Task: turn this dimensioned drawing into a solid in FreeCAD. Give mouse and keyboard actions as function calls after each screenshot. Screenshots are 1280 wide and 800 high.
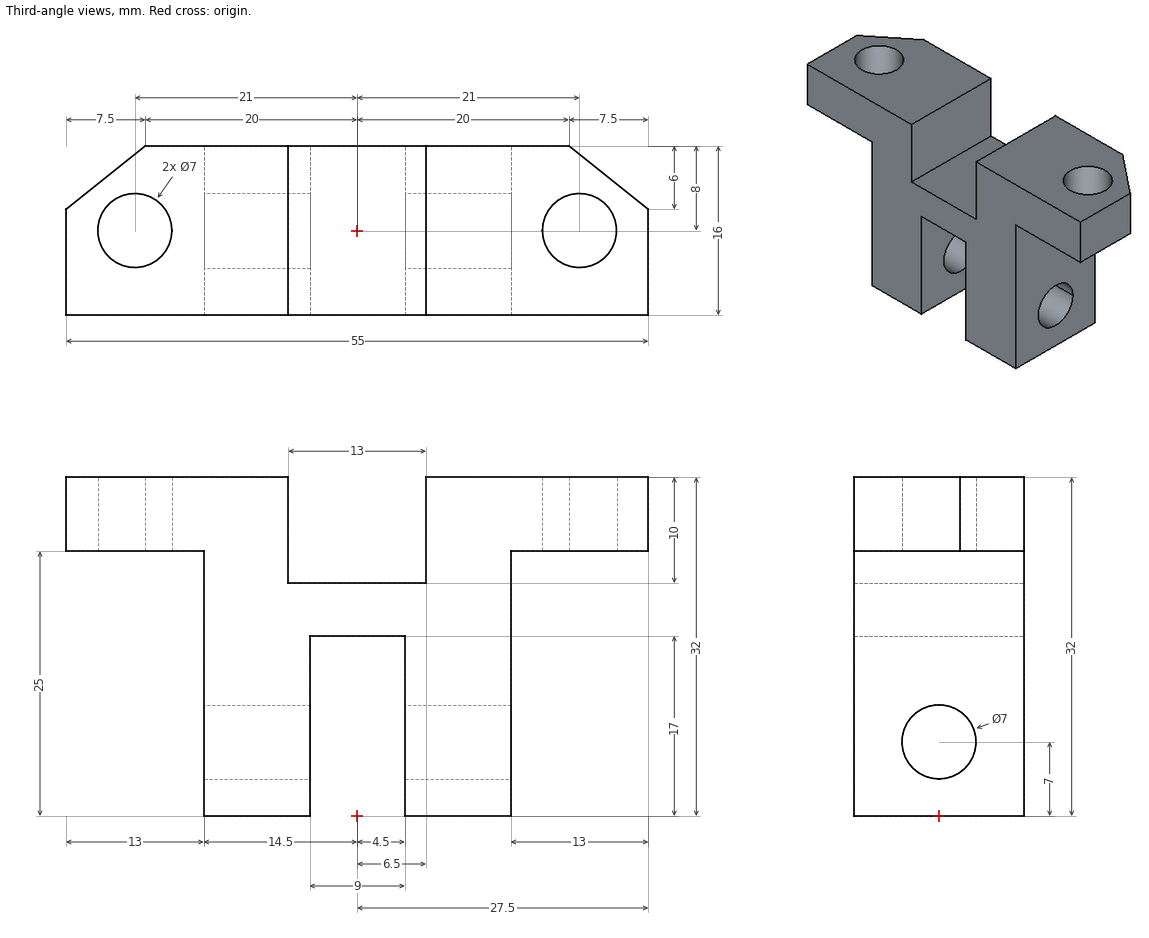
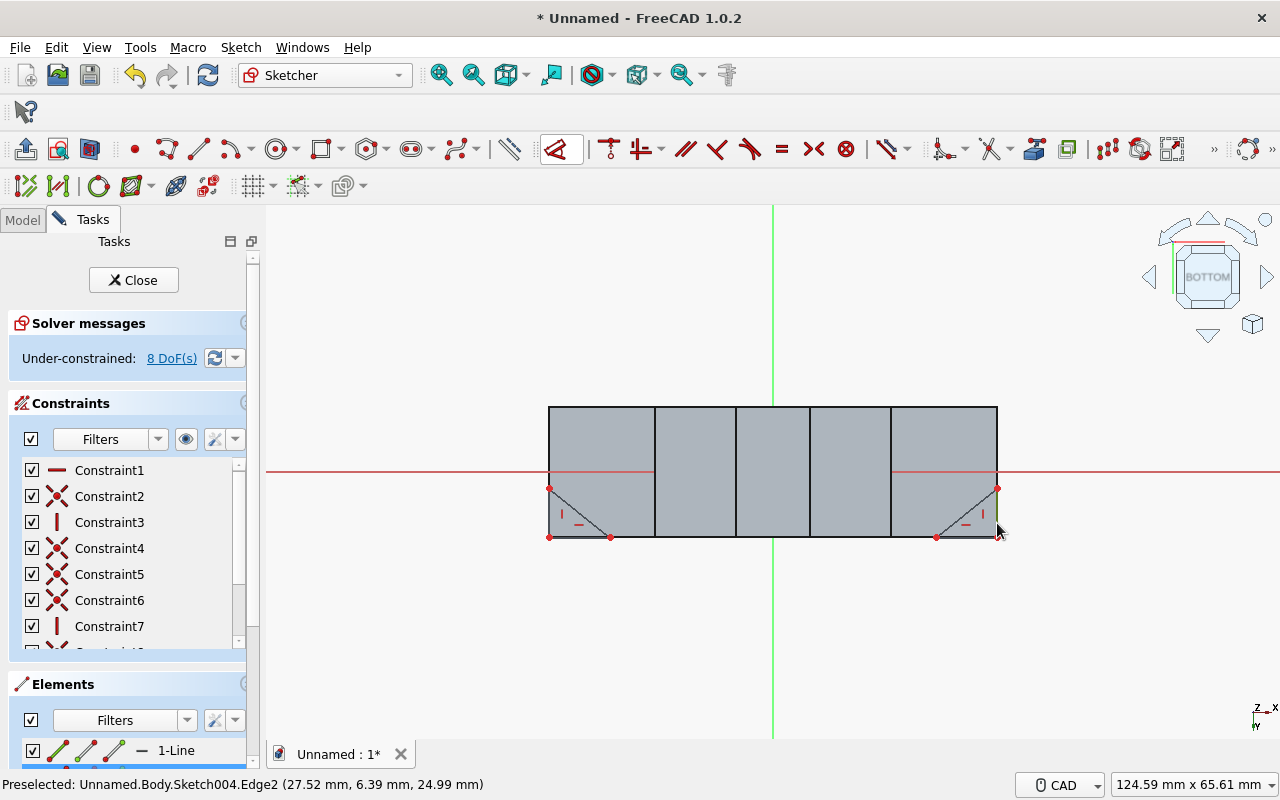
click(578, 150)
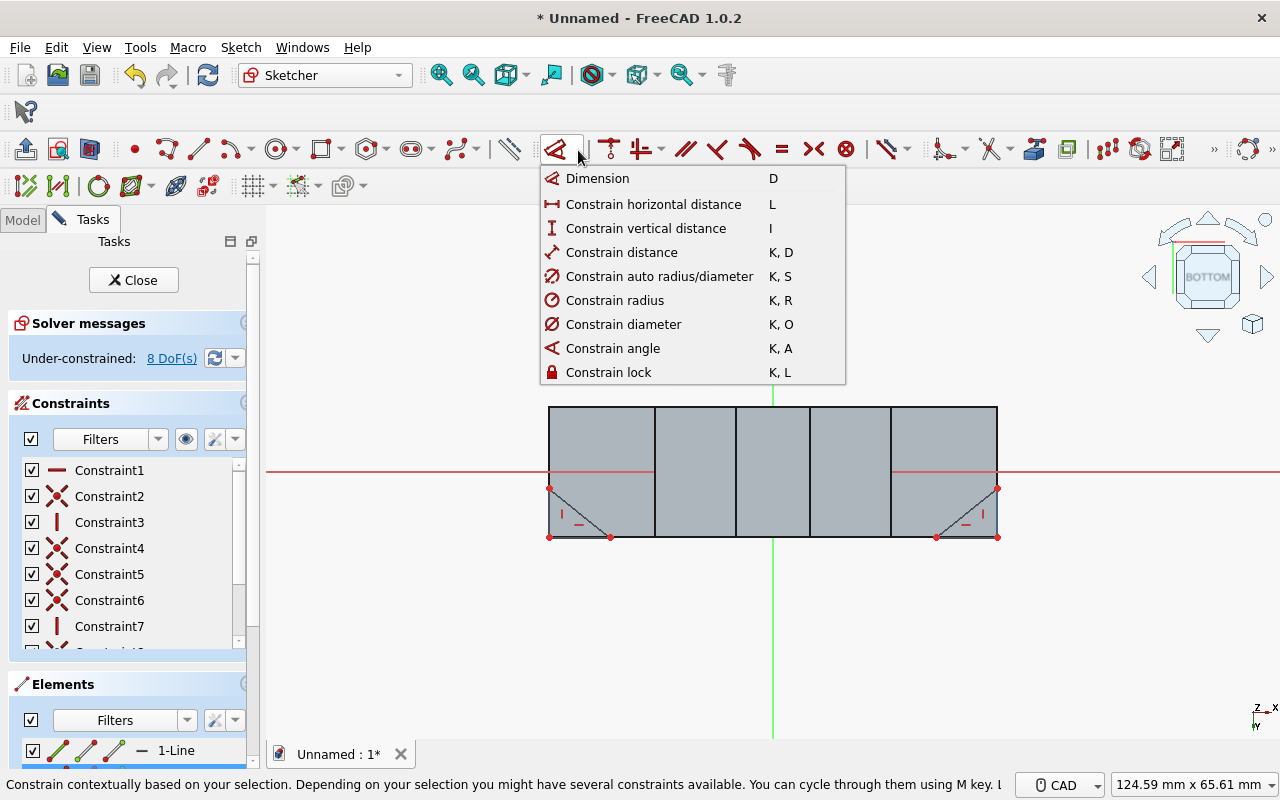
click(693, 228)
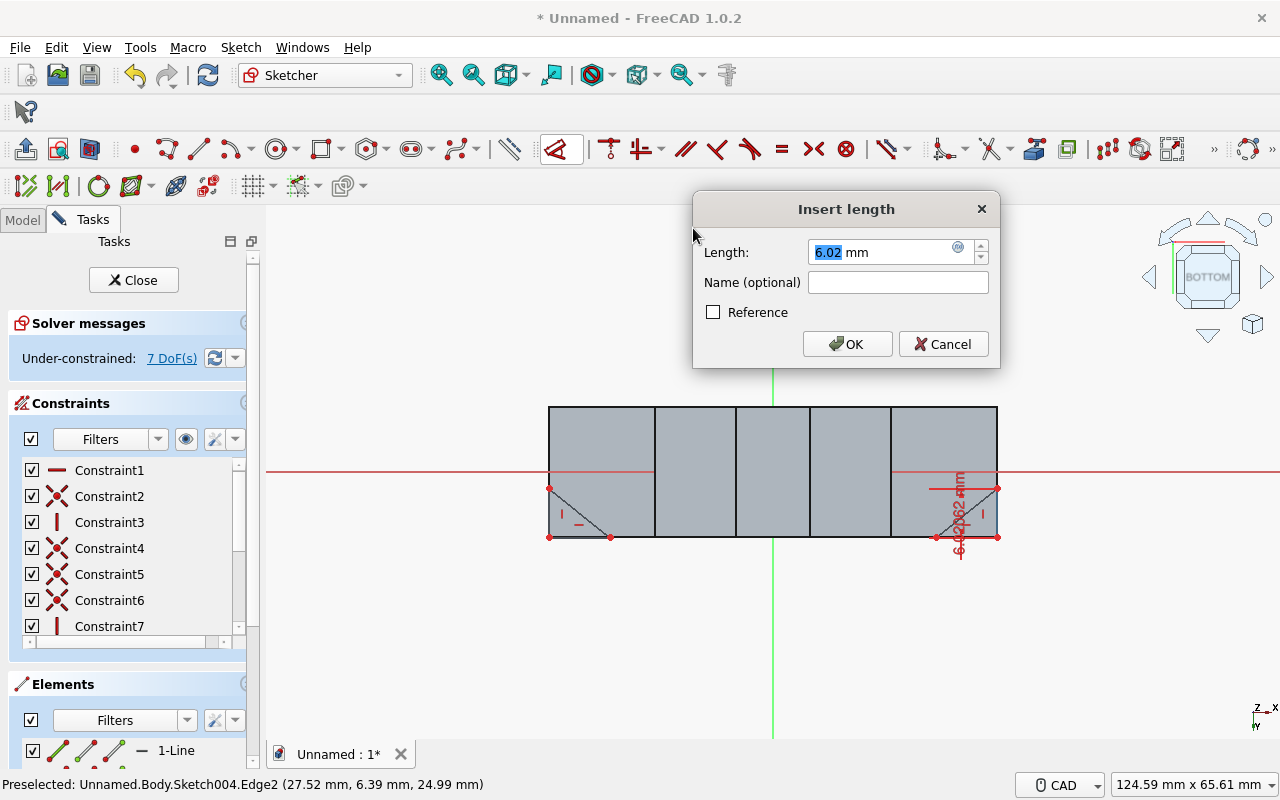
text(6)
key(Return)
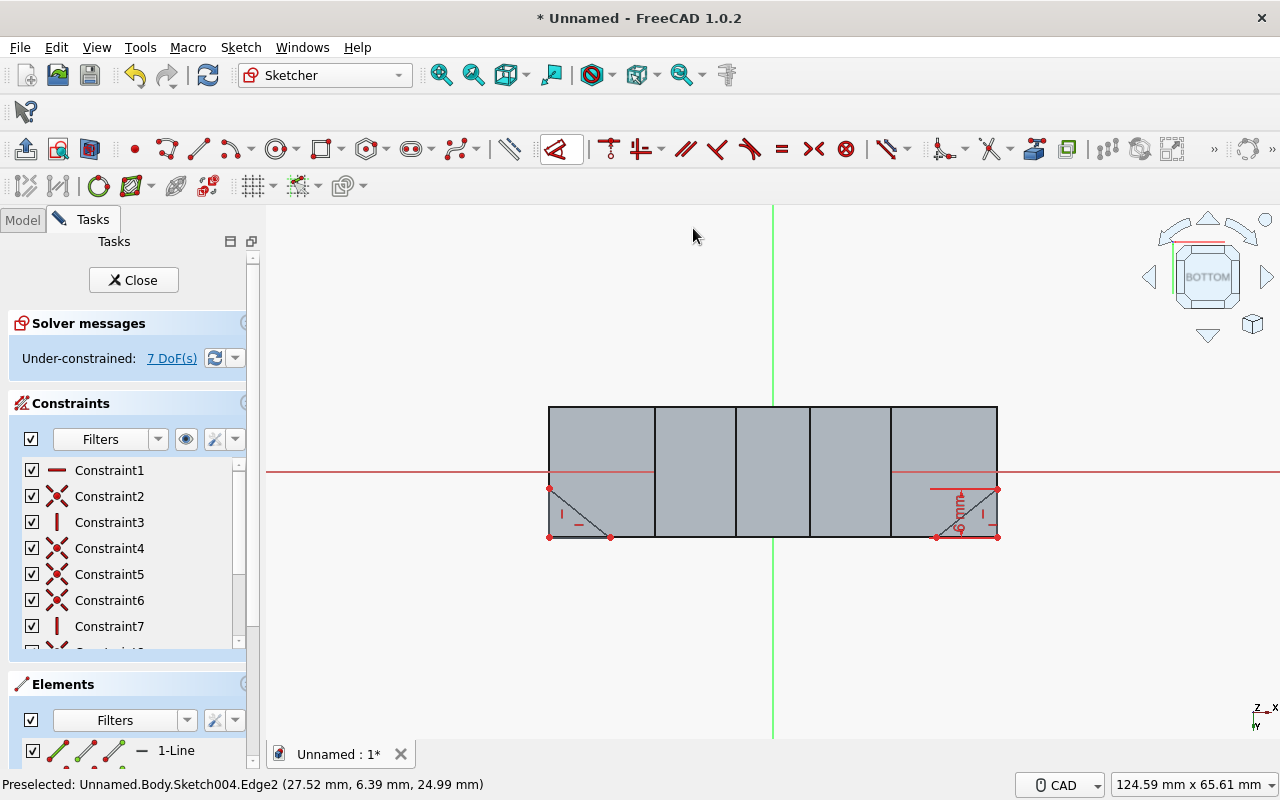
click(549, 504)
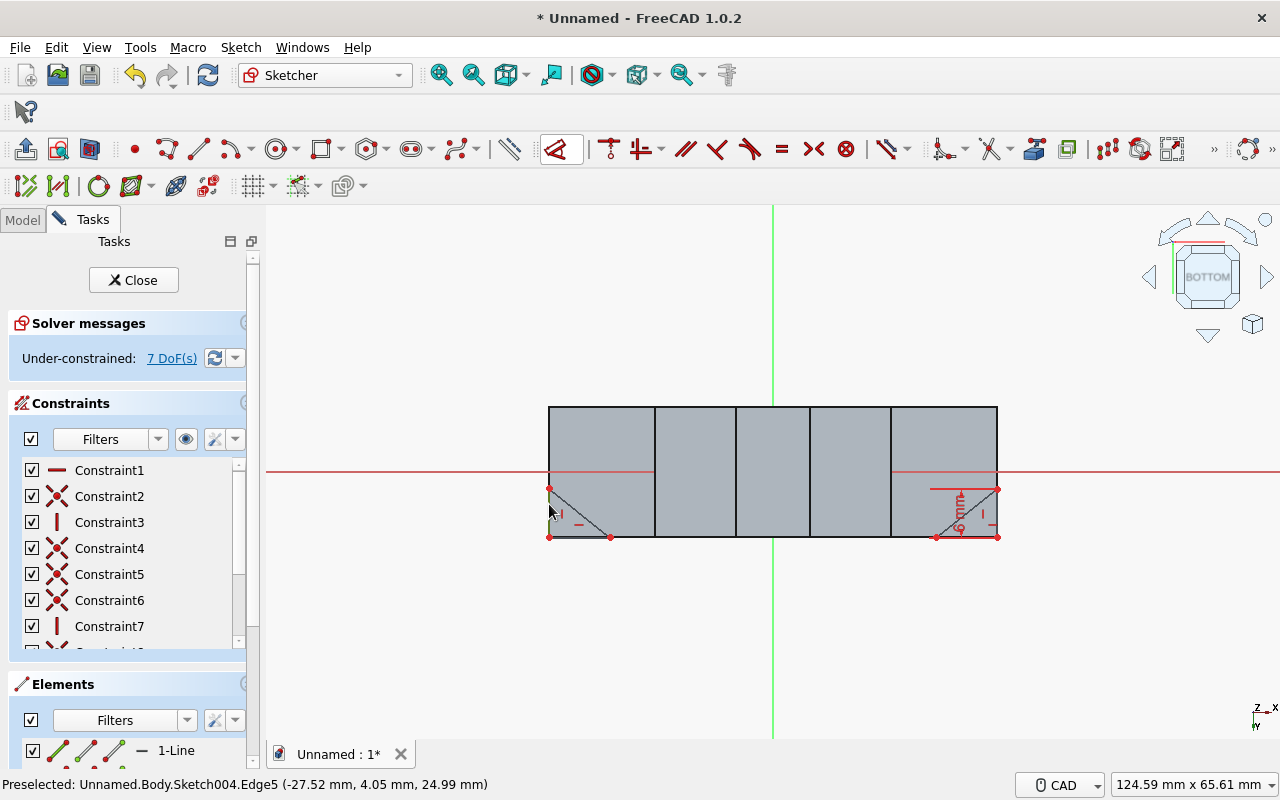
click(578, 150)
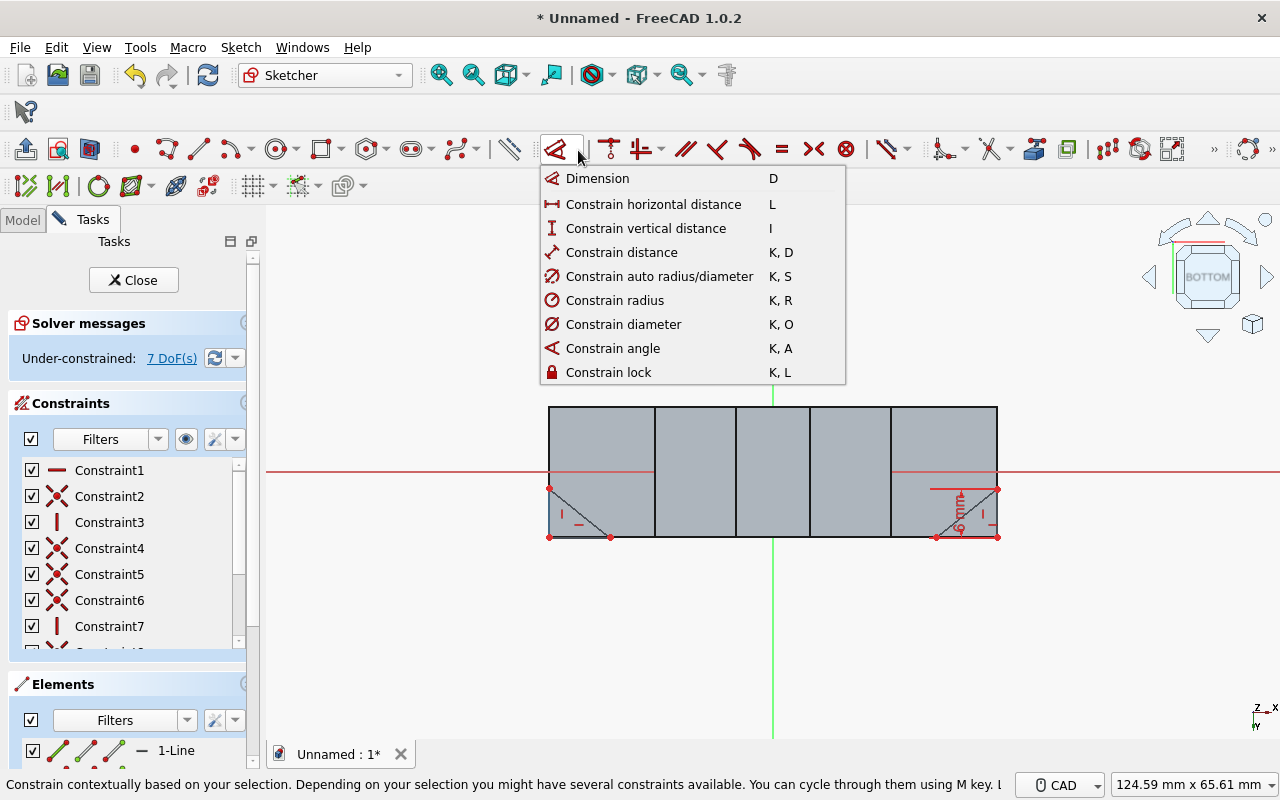
click(693, 228)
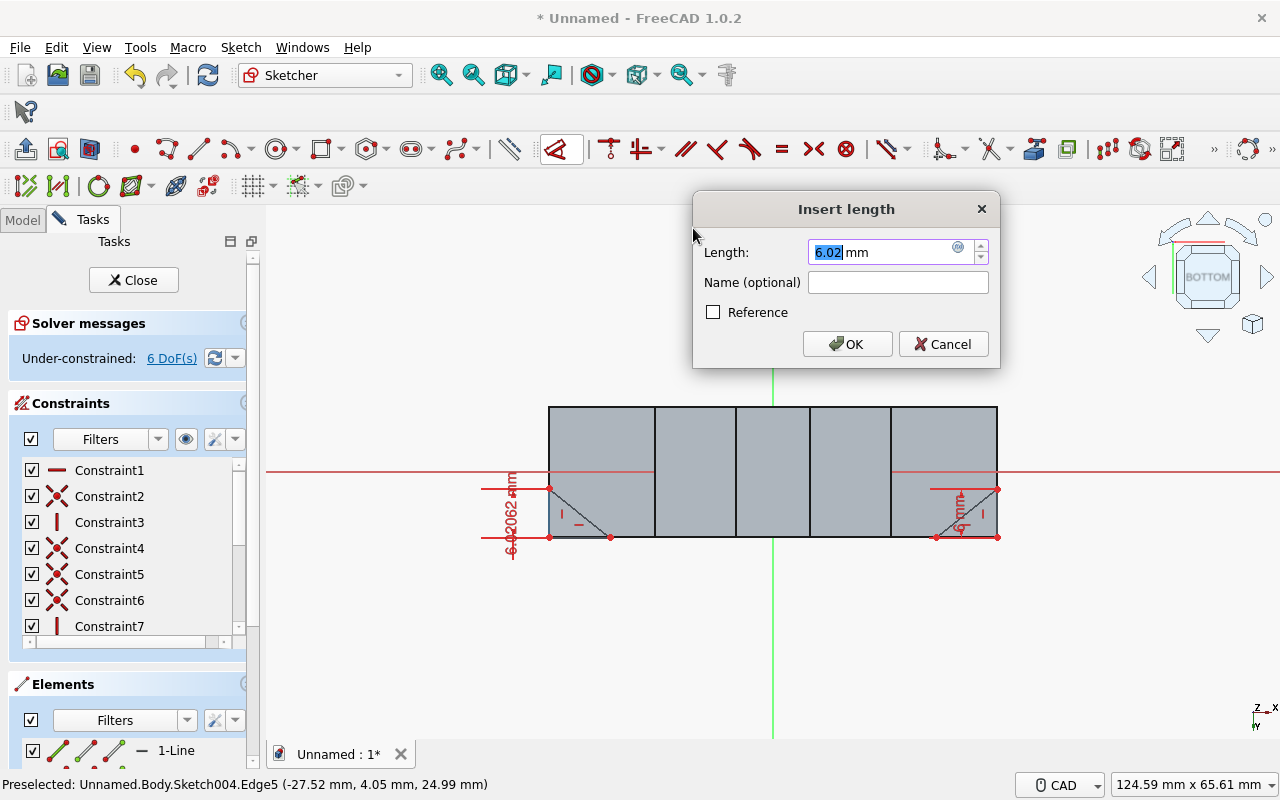
text(6)
key(Return)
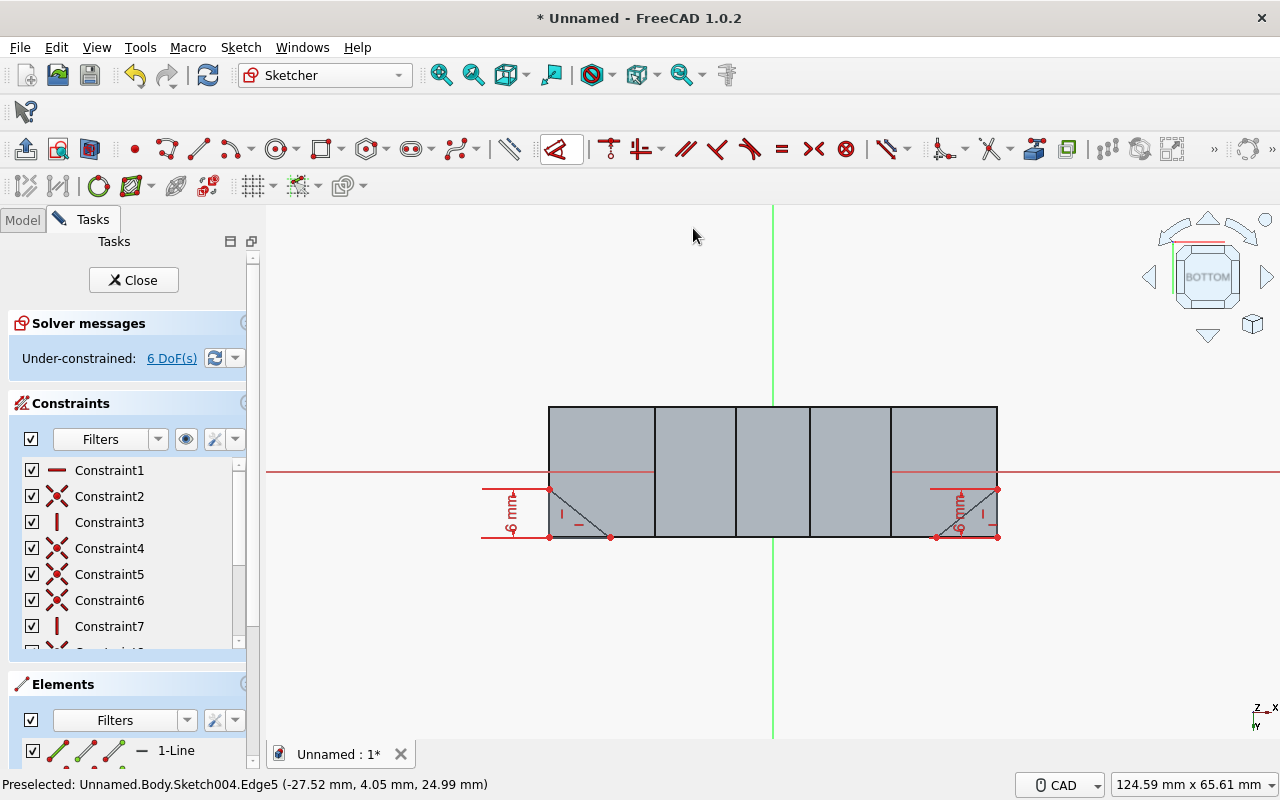
click(936, 538)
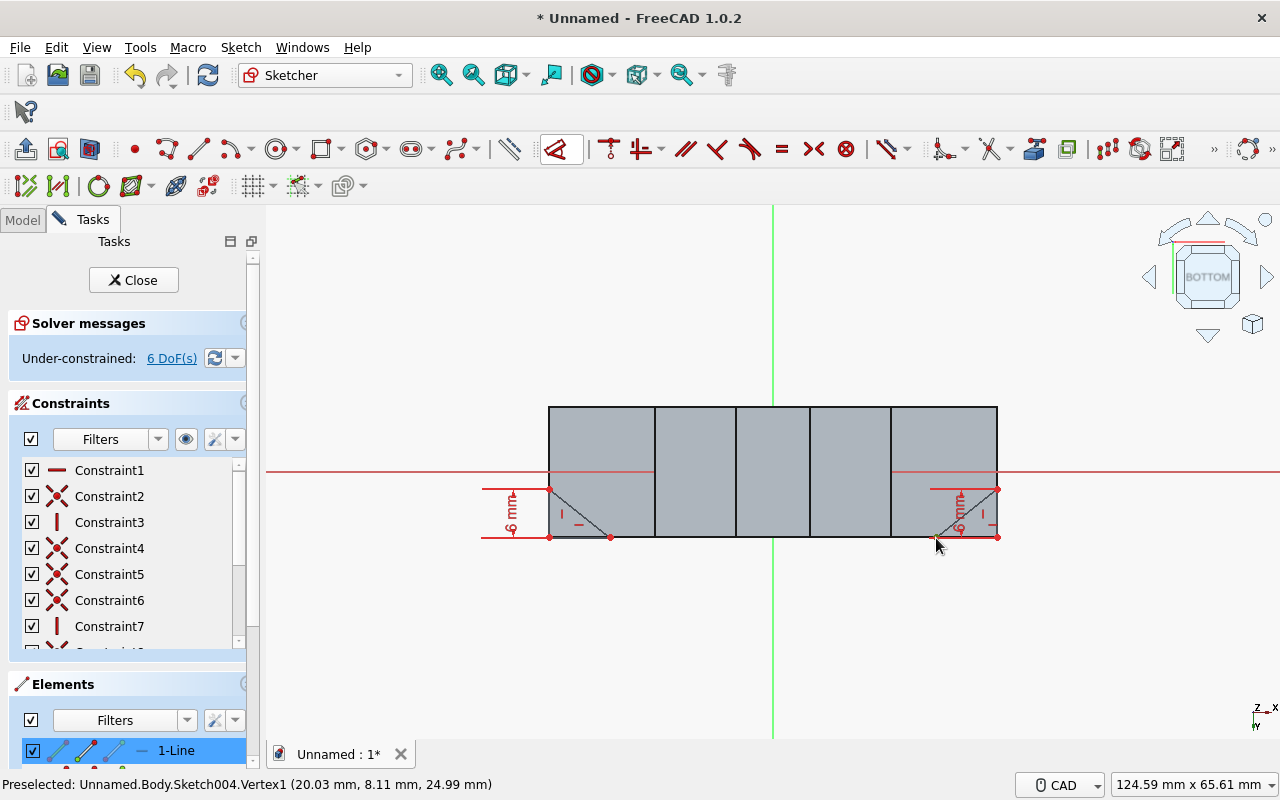
key(i)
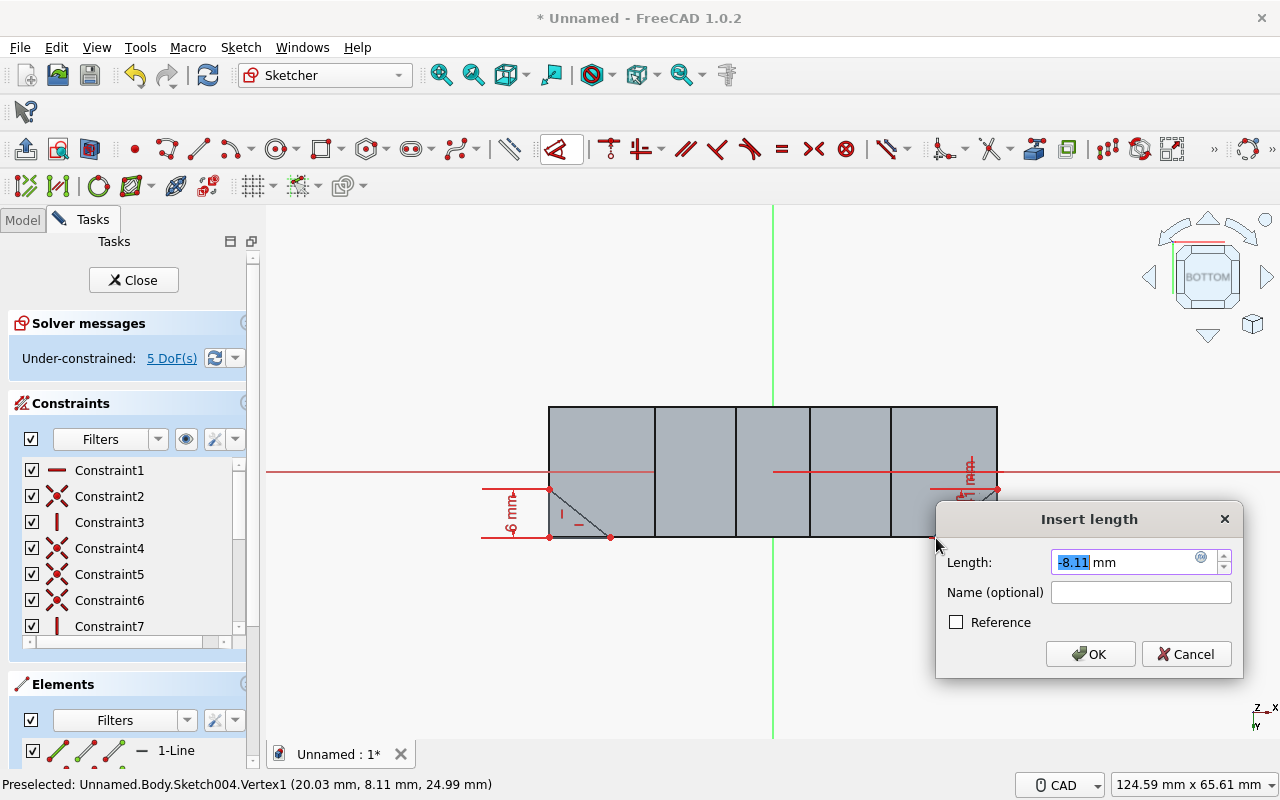
text(-8)
key(Return)